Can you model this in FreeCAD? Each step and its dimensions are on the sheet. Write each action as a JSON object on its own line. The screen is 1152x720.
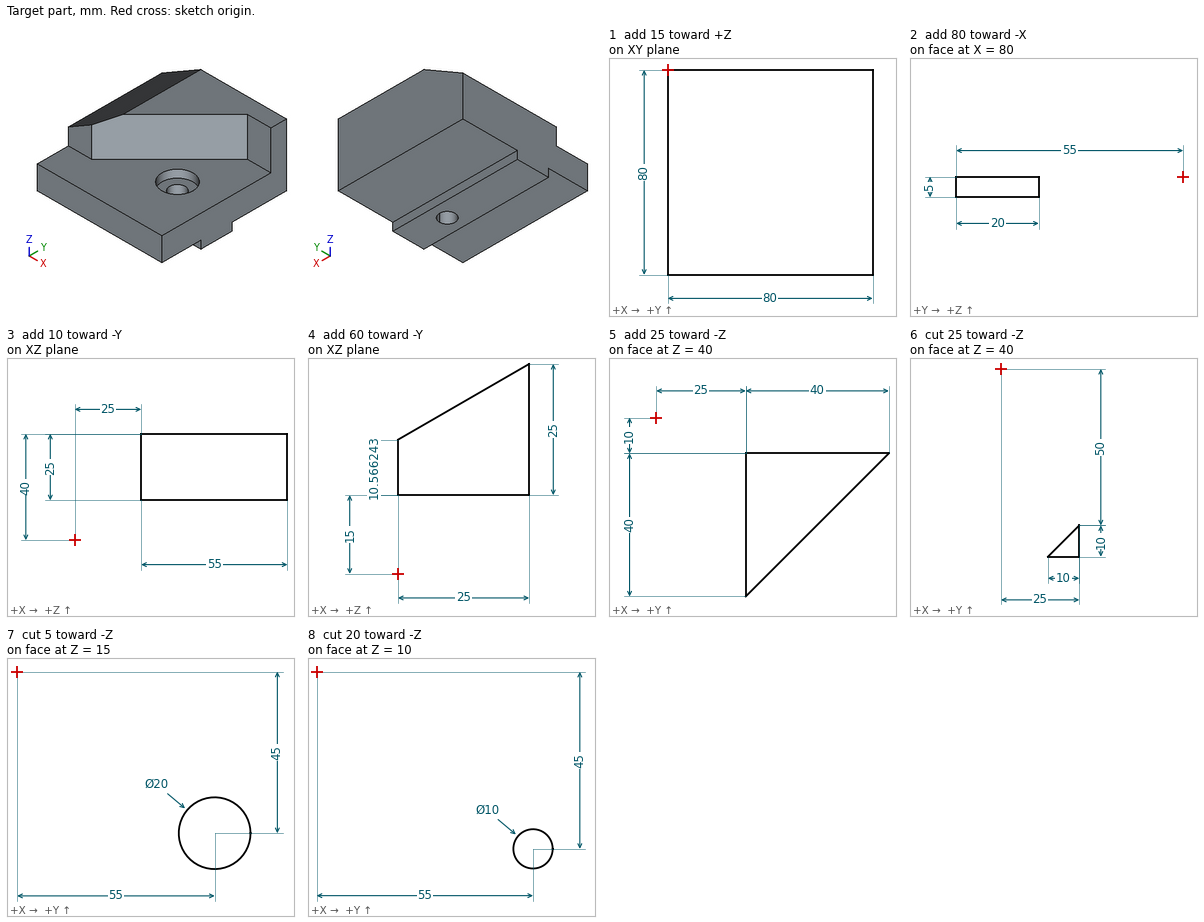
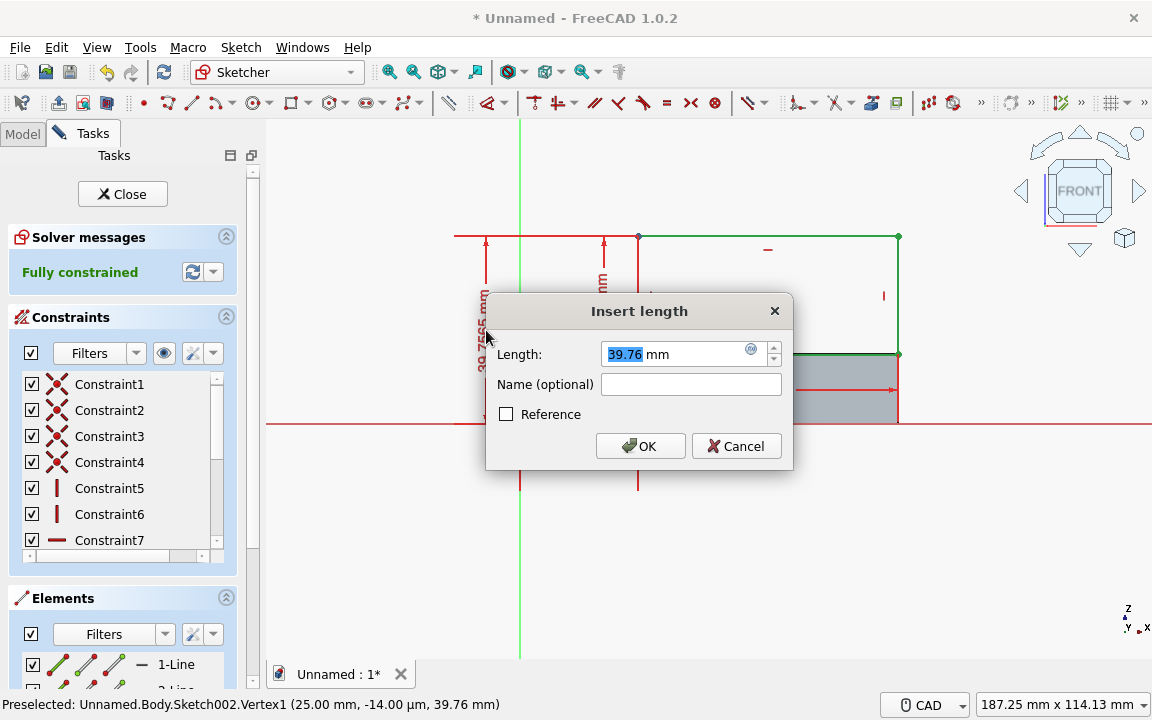
{"action": "type", "text": "40"}
{"action": "key", "text": "Return"}
{"action": "key", "text": "Escape"}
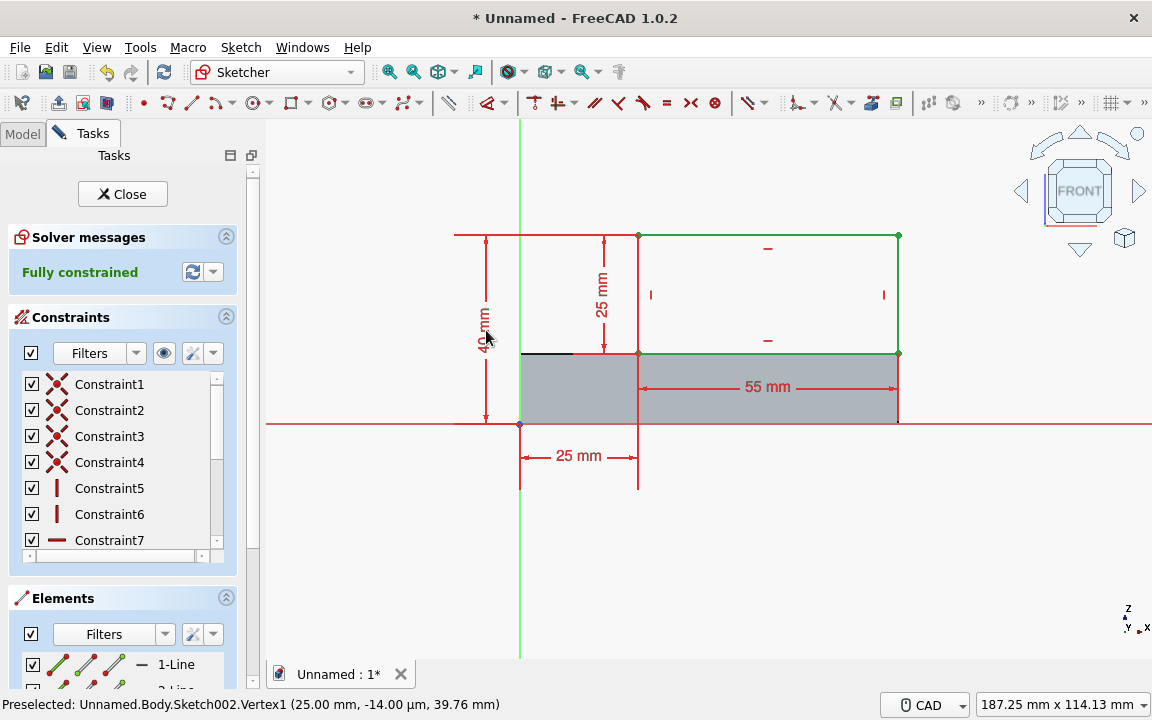
{"action": "left_click", "coordinate": [123, 194]}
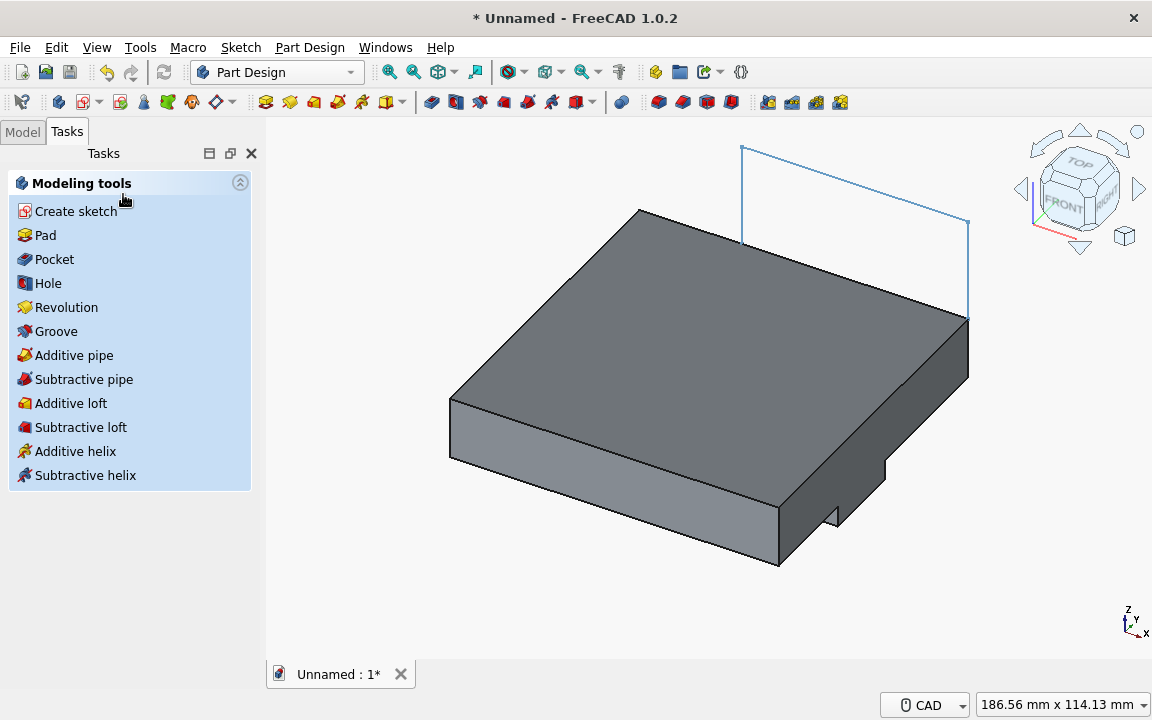
{"action": "left_click", "coordinate": [266, 102]}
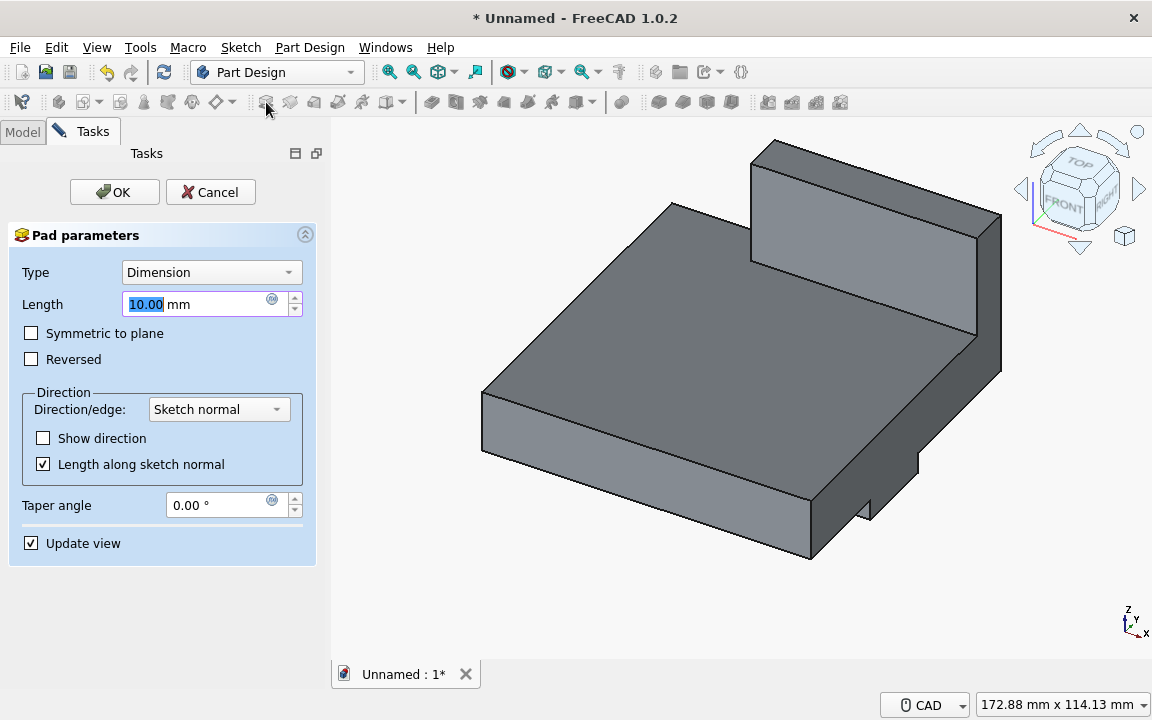
{"action": "type", "text": "10"}
{"action": "key", "text": "Tab"}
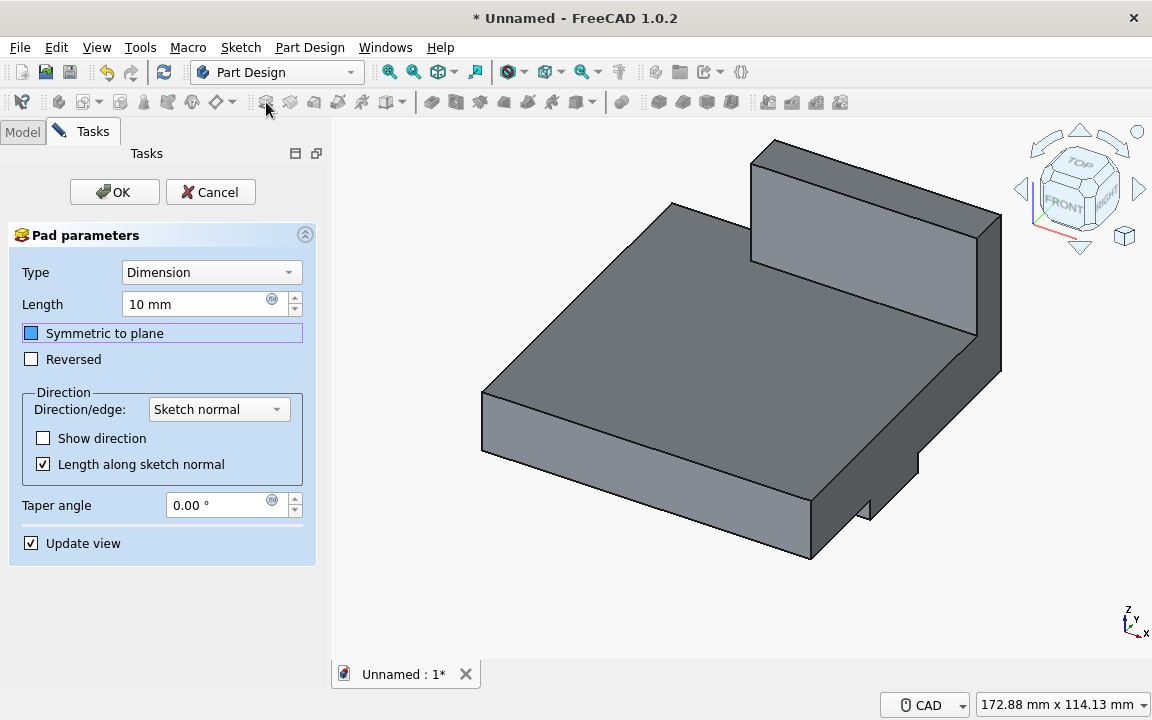
{"action": "left_click", "coordinate": [115, 192]}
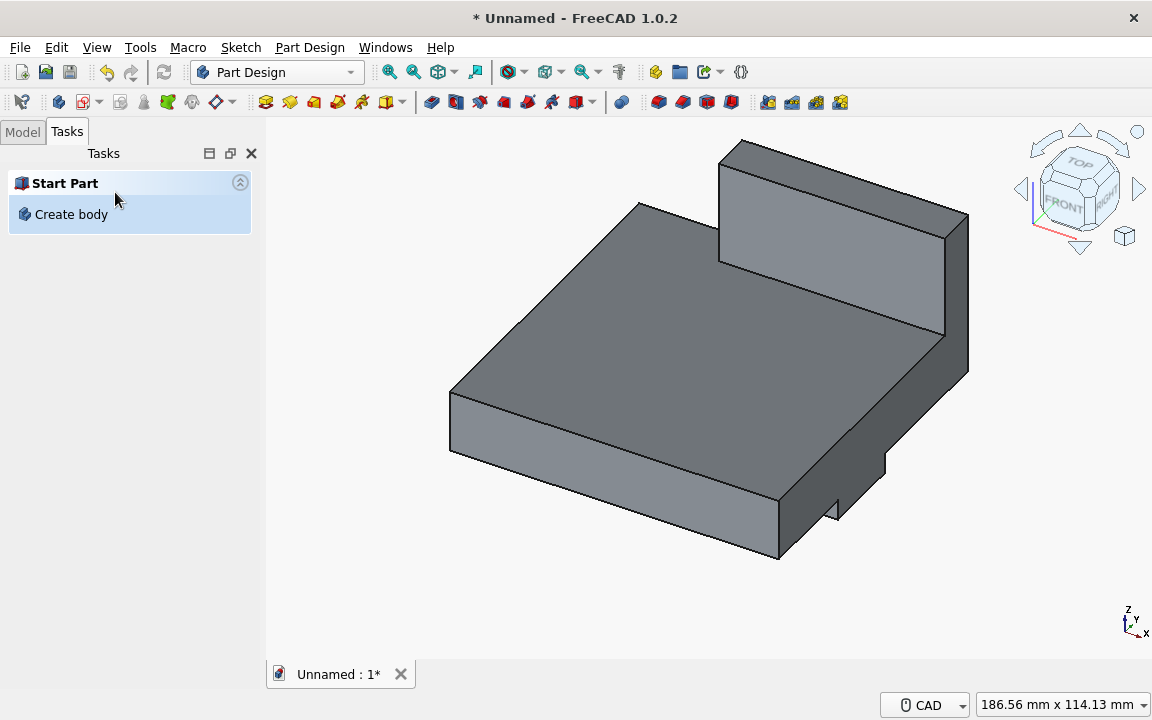
{"action": "left_click", "coordinate": [390, 72]}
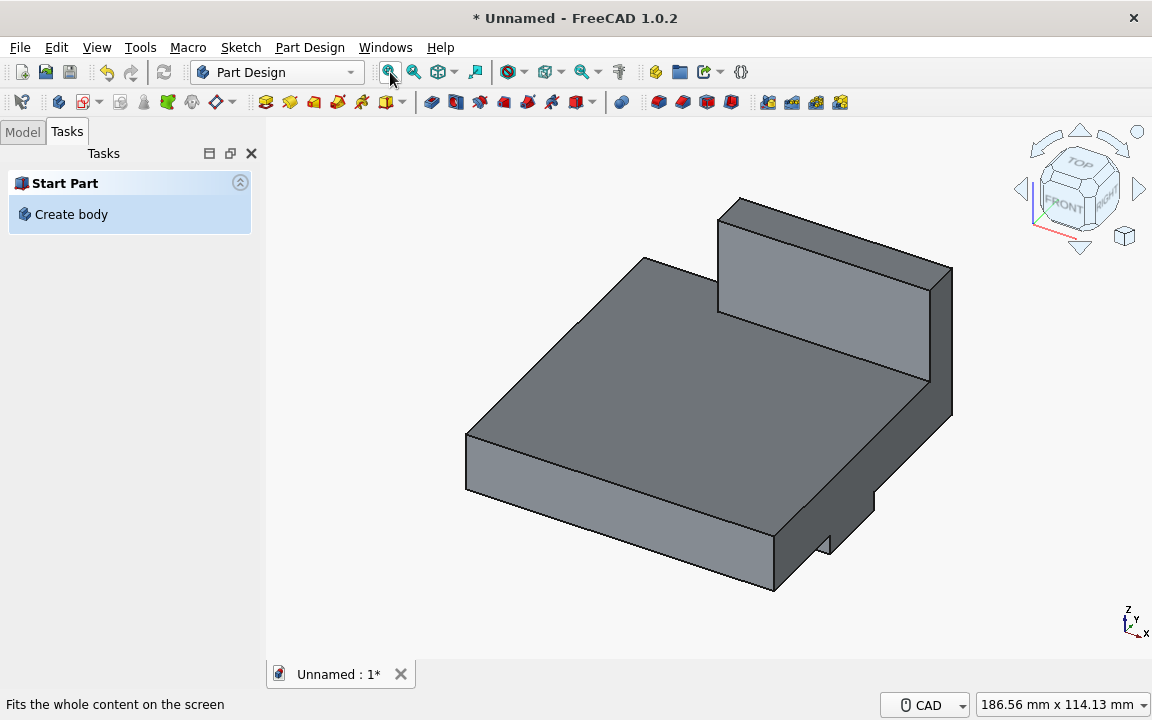
{"action": "left_click", "coordinate": [84, 102]}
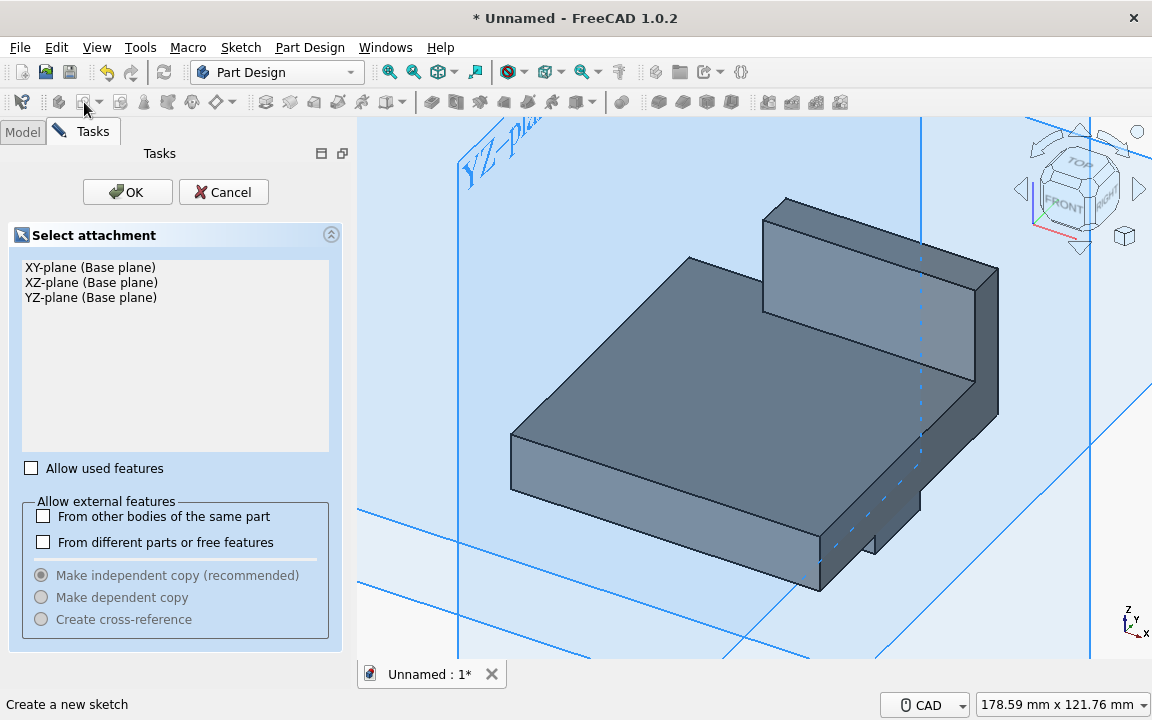
{"action": "left_click", "coordinate": [82, 282]}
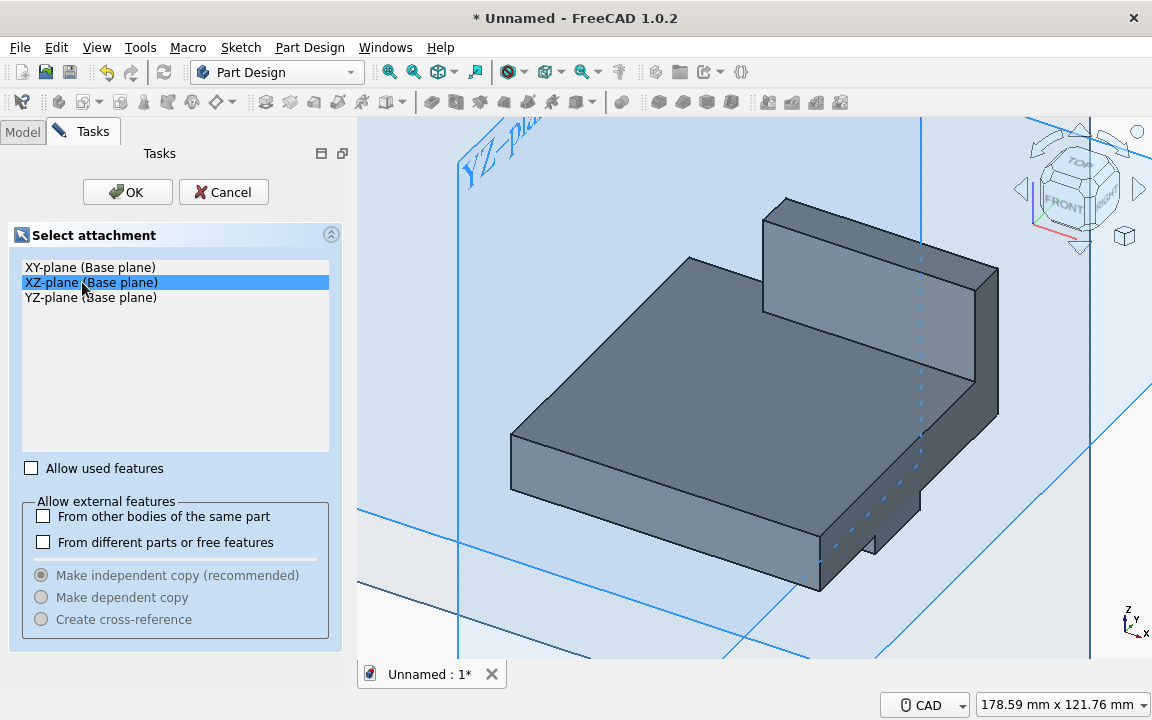
{"action": "left_click", "coordinate": [128, 192]}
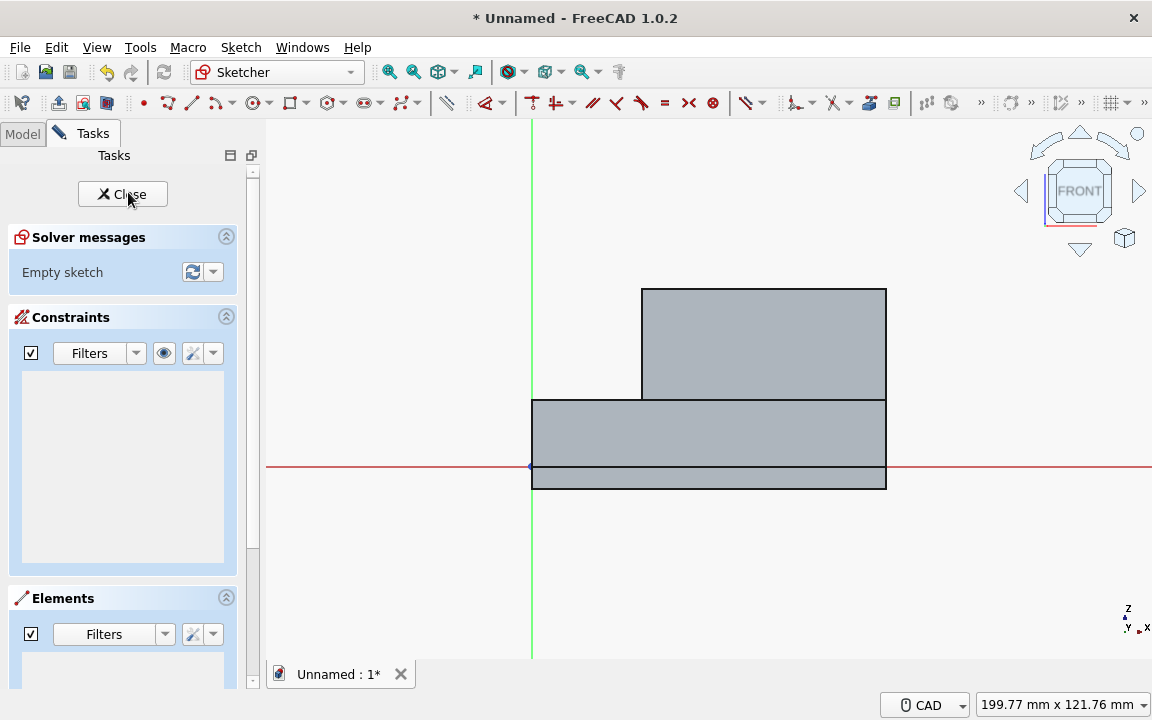
{"action": "left_click", "coordinate": [108, 104]}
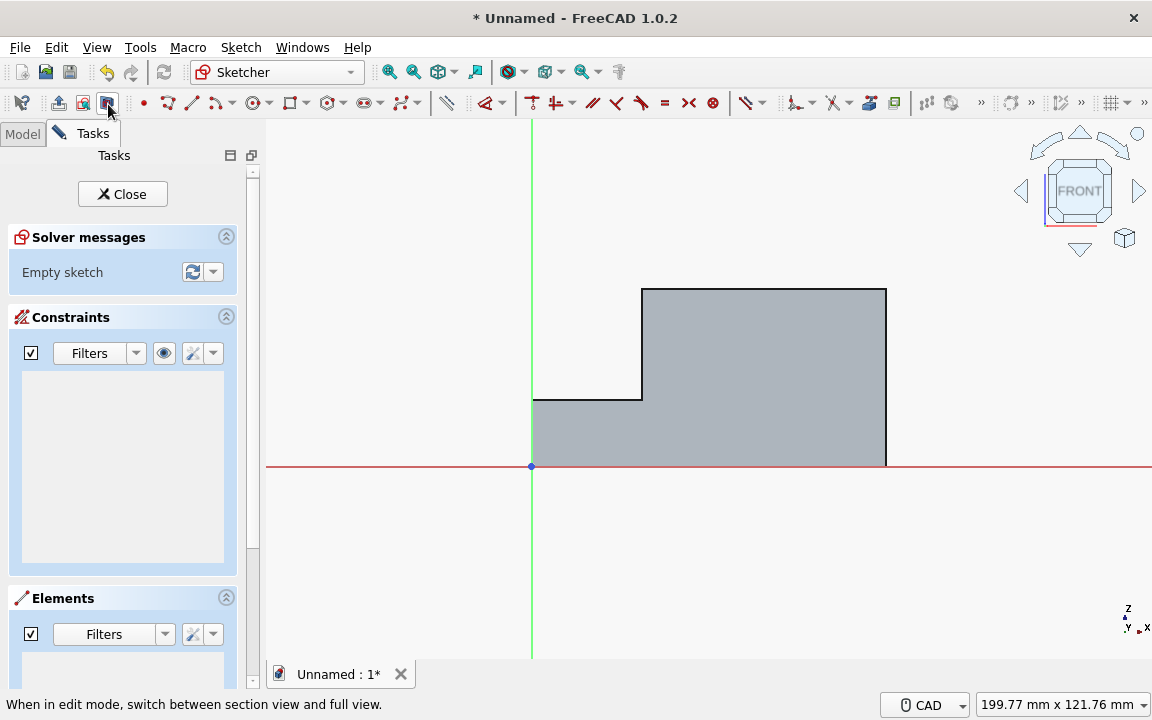
{"action": "scroll", "coordinate": [522, 364], "scroll_direction": "up", "scroll_amount": 3}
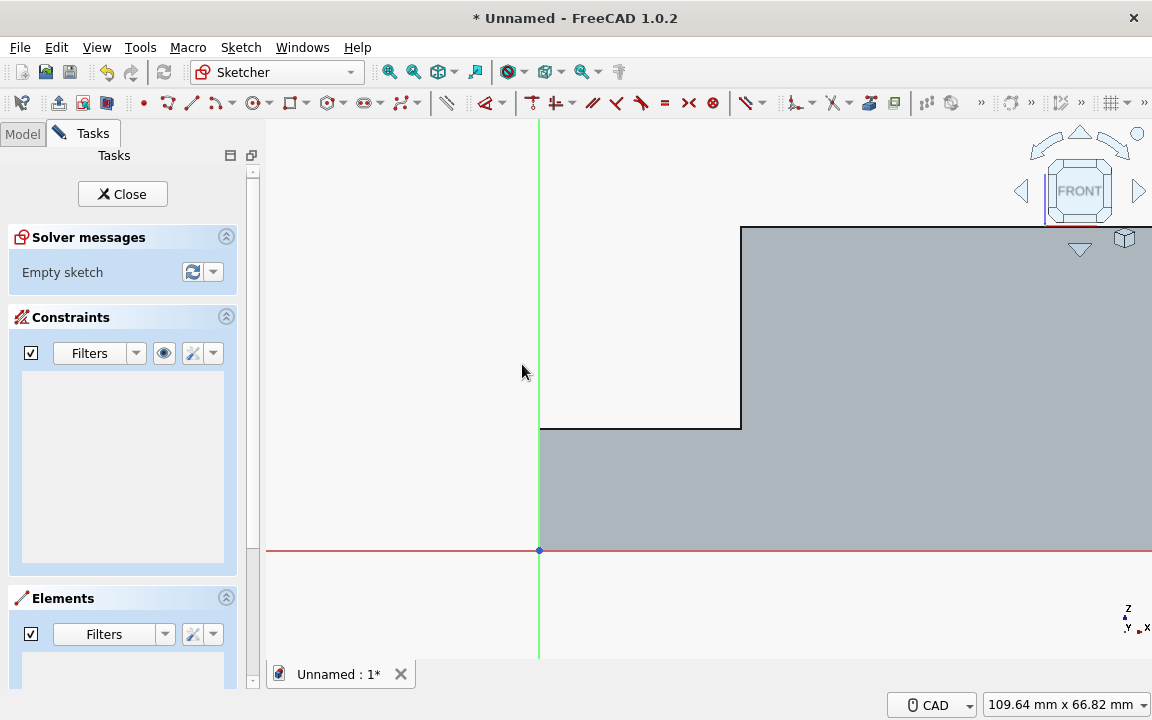
{"action": "left_click", "coordinate": [168, 104]}